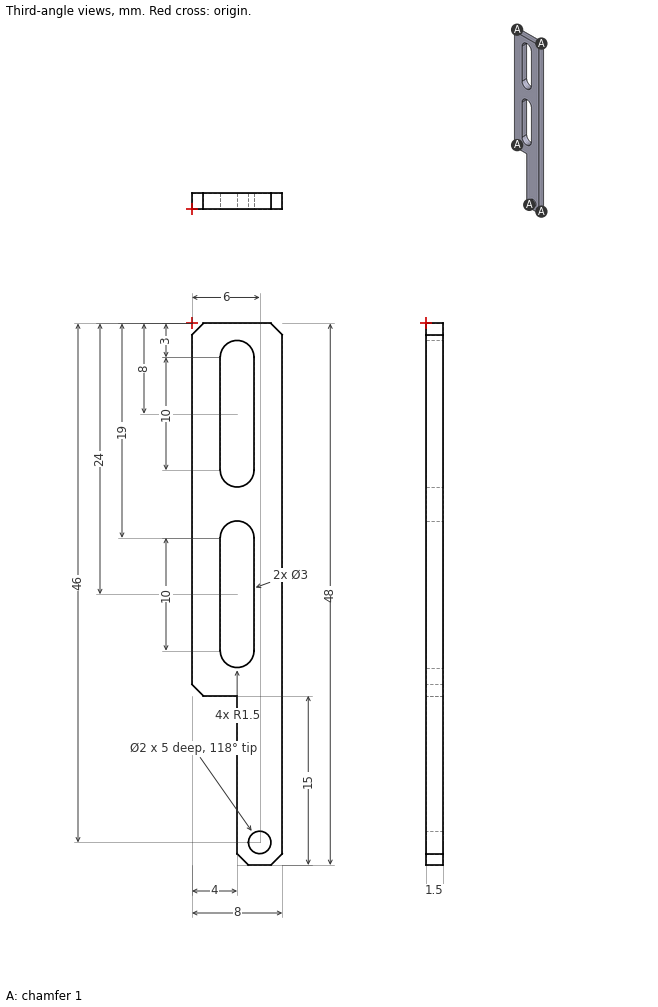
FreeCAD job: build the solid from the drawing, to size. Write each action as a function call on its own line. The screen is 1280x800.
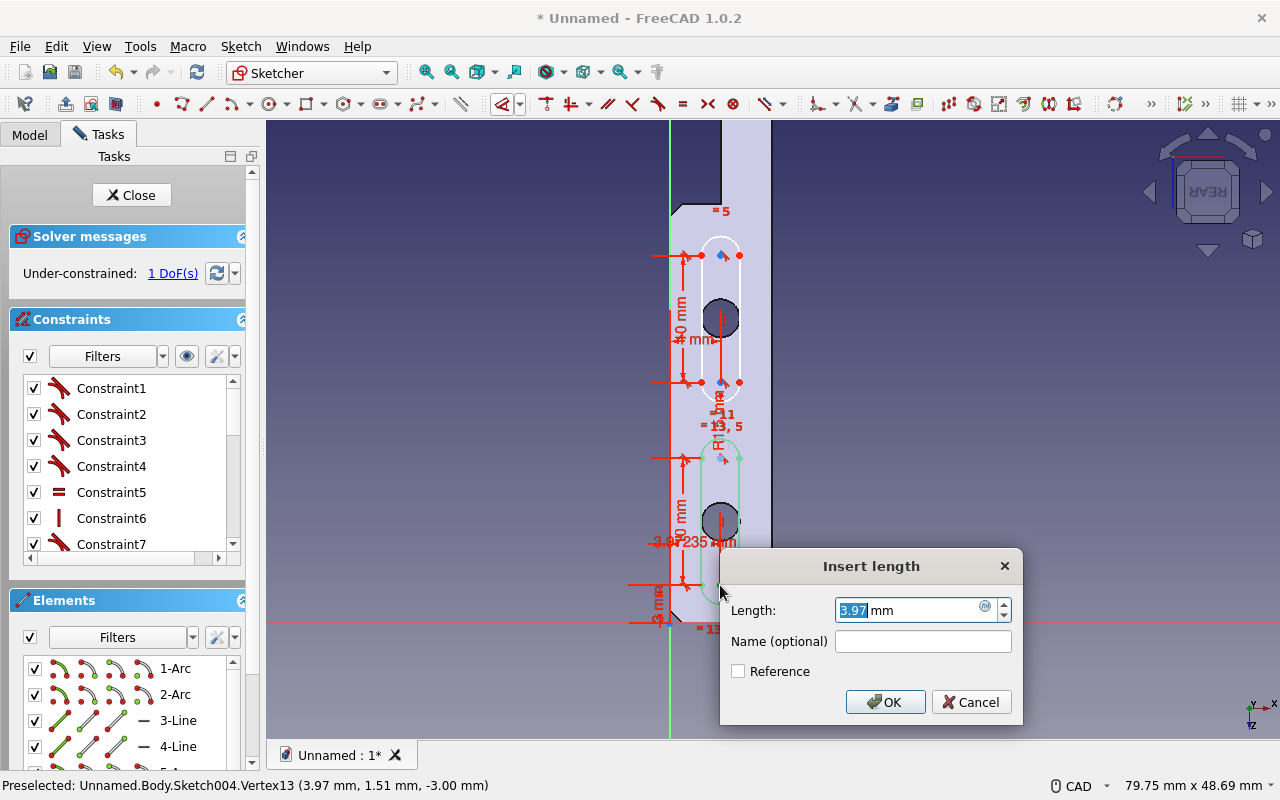
text(4)
key(Return)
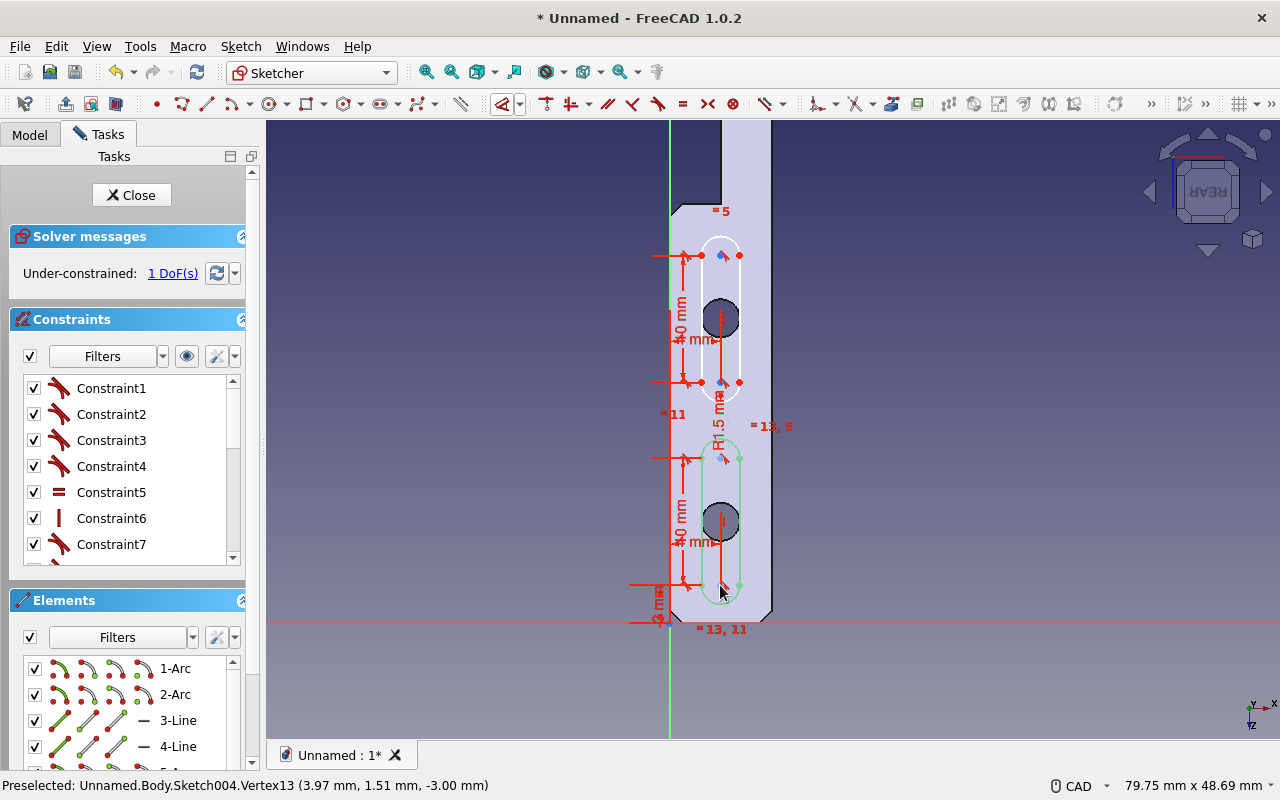
click(702, 383)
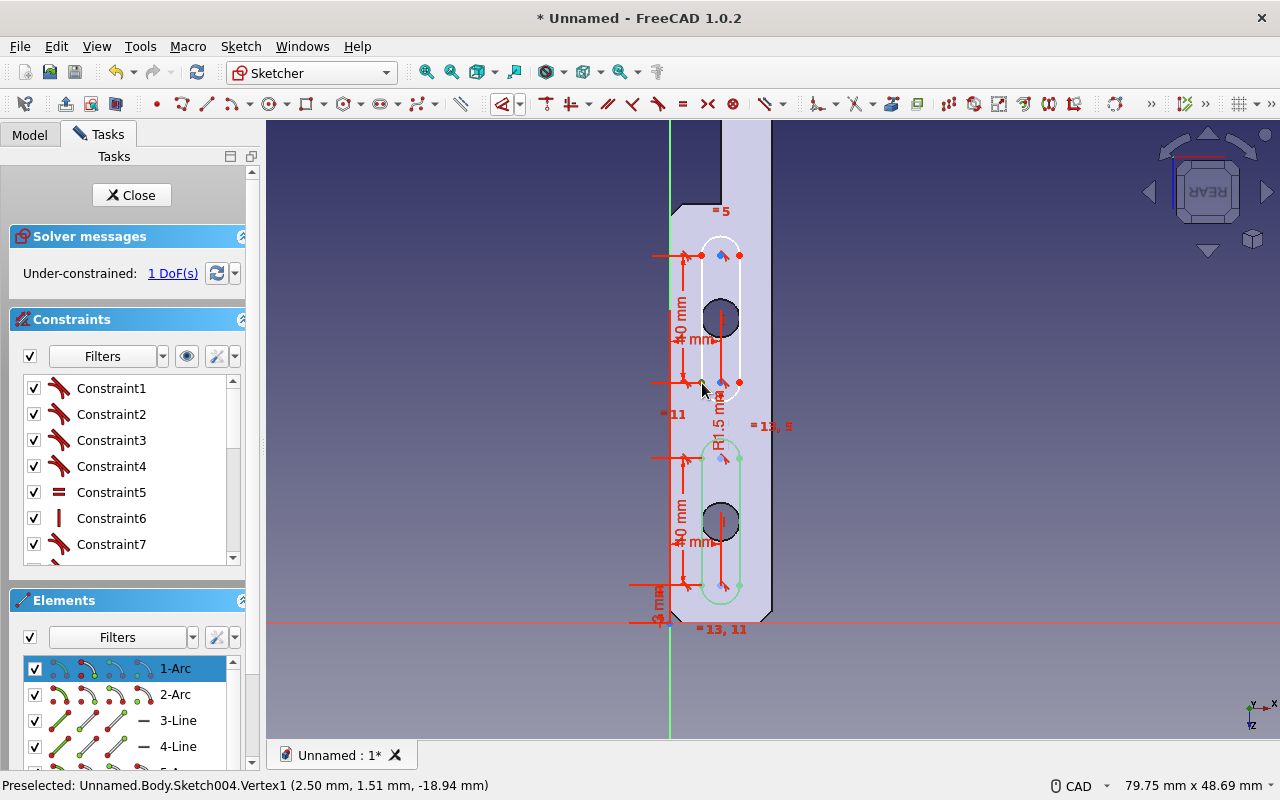
key(i)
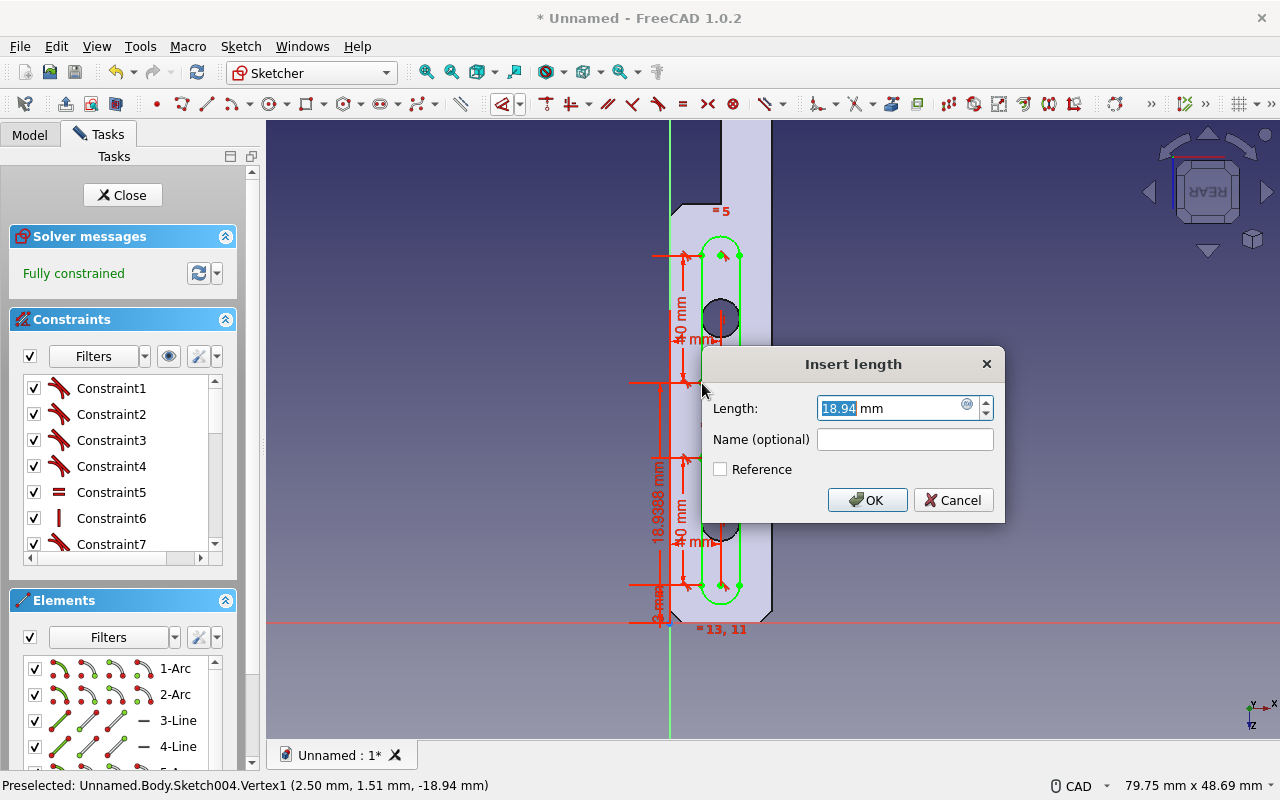
text(19)
key(Return)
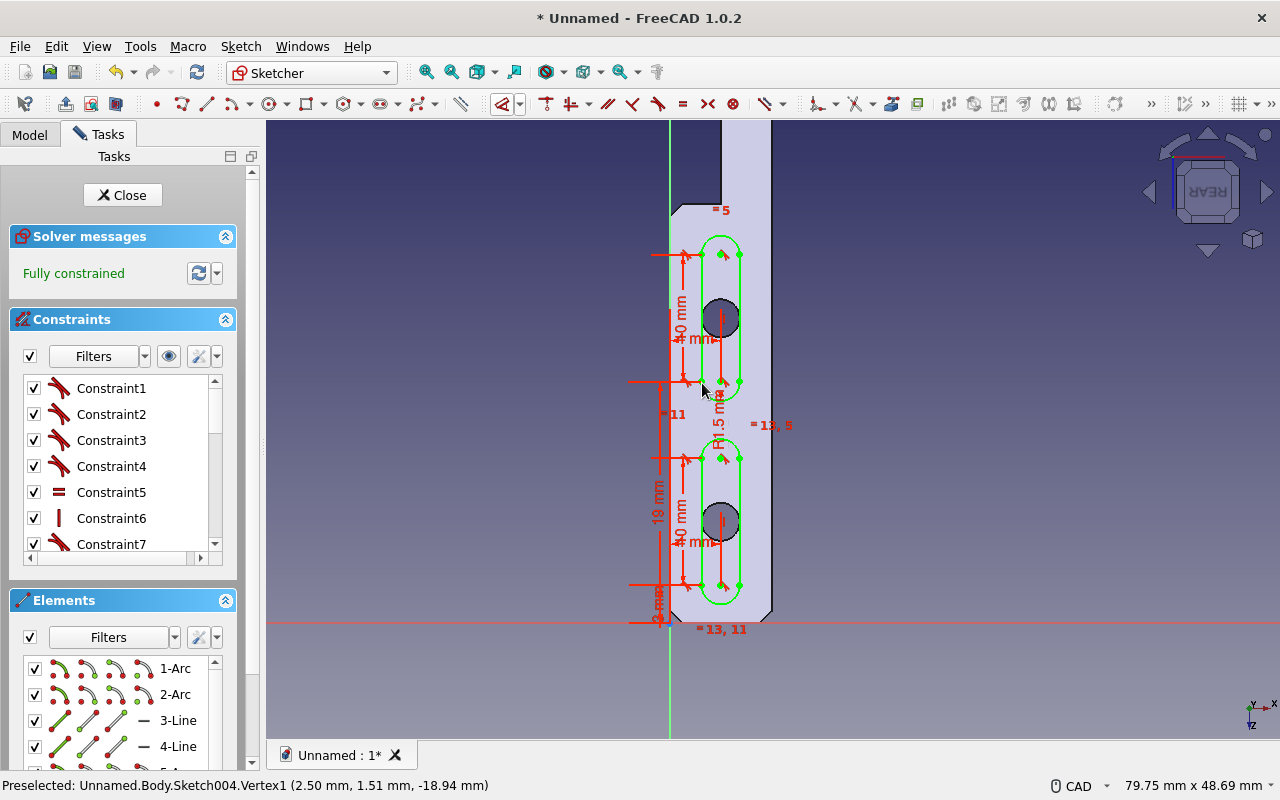
click(123, 195)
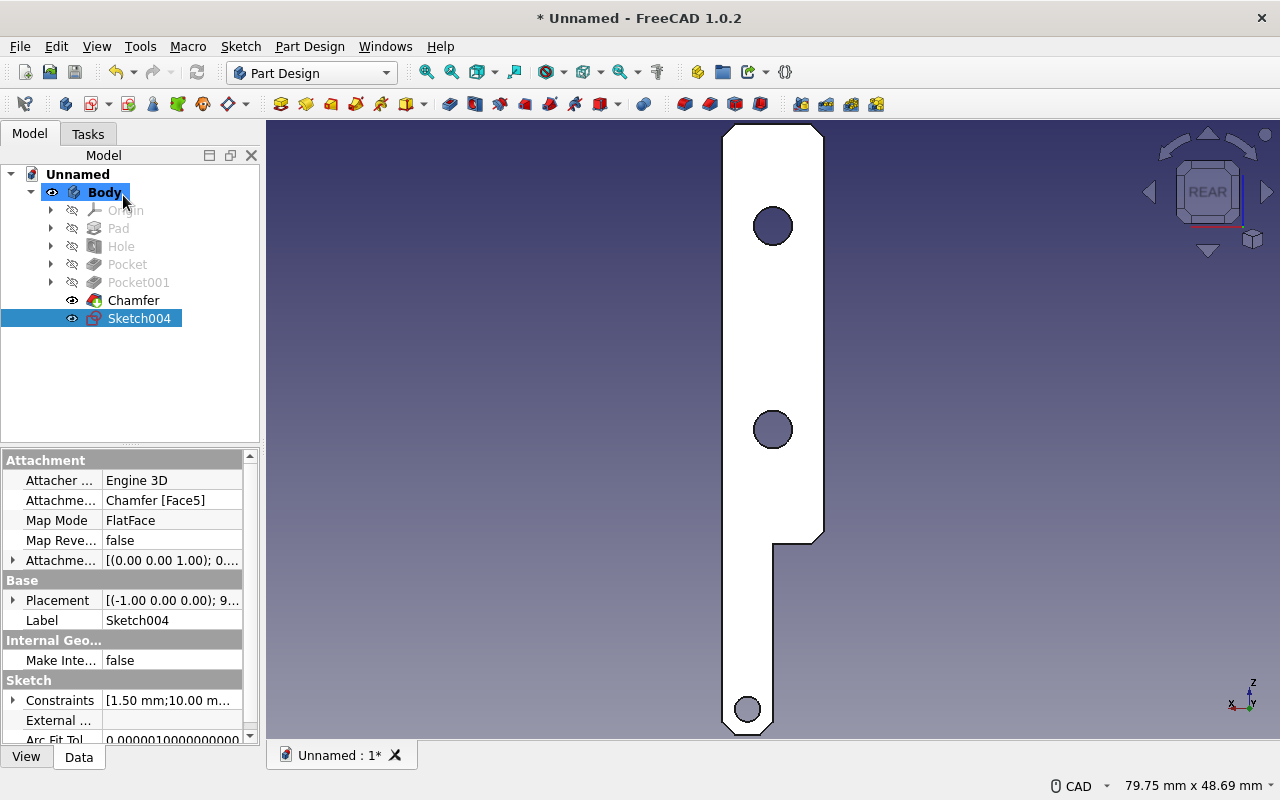
click(450, 104)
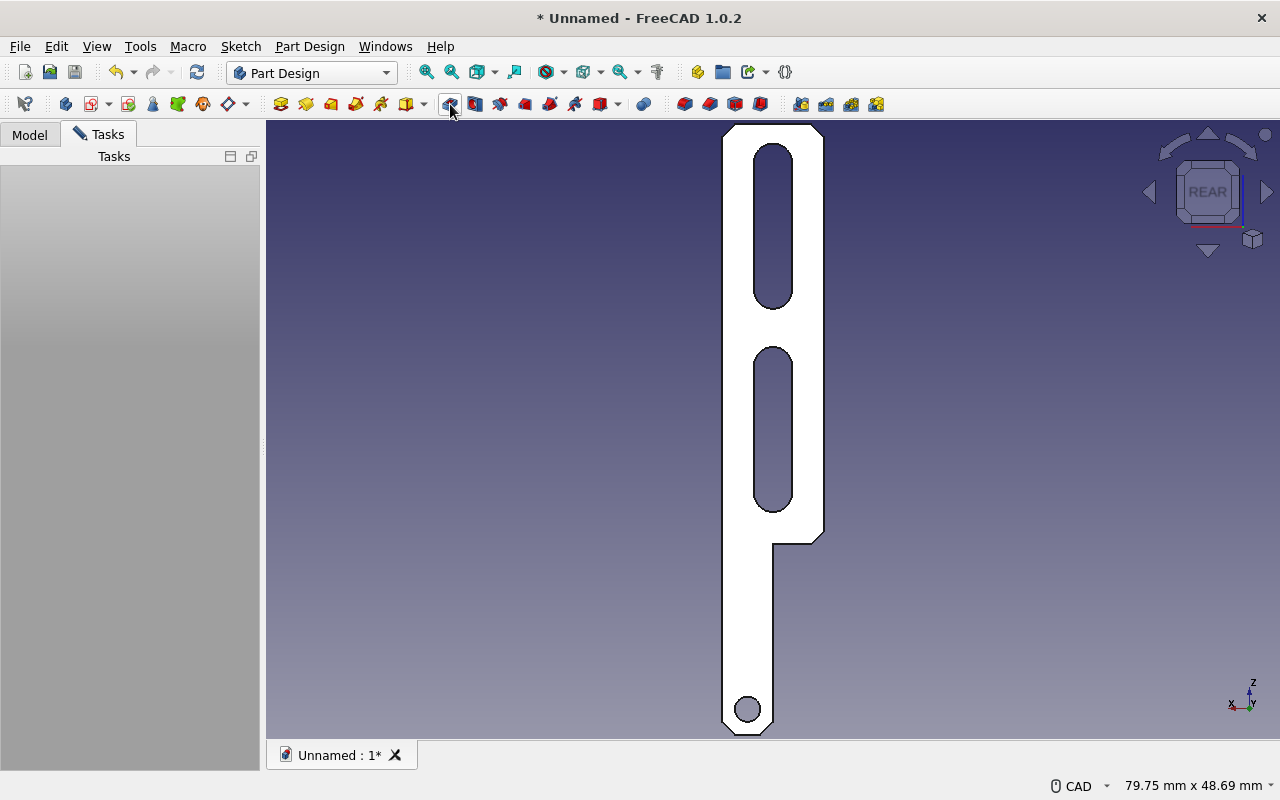
text(10)
key(Tab)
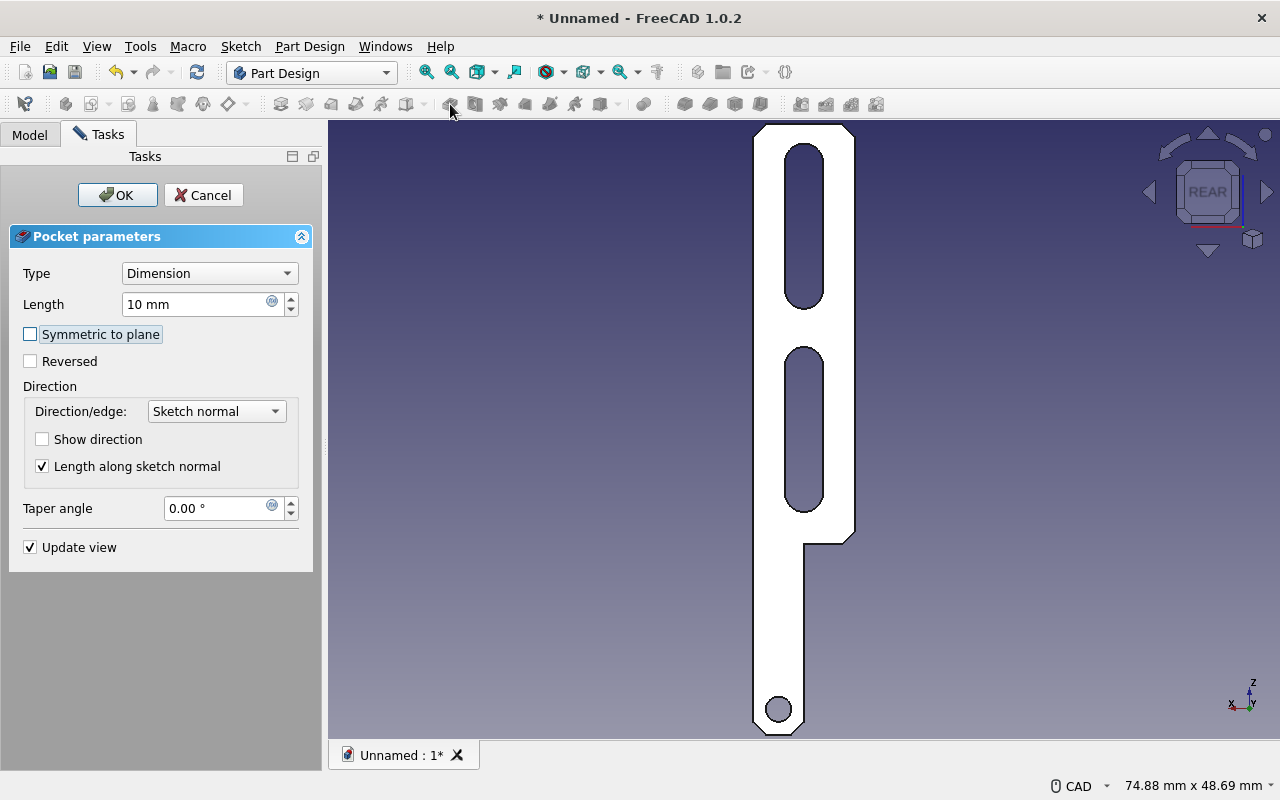
click(118, 195)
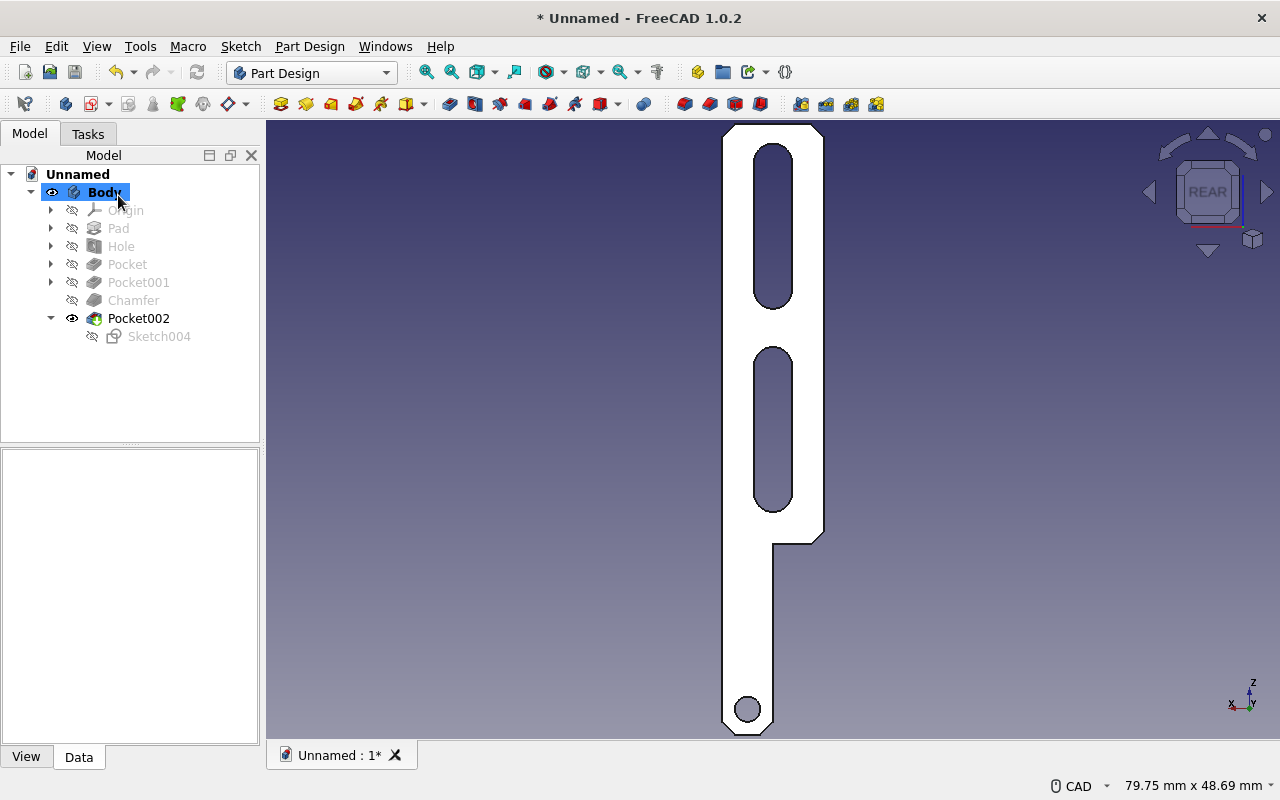
key(0)